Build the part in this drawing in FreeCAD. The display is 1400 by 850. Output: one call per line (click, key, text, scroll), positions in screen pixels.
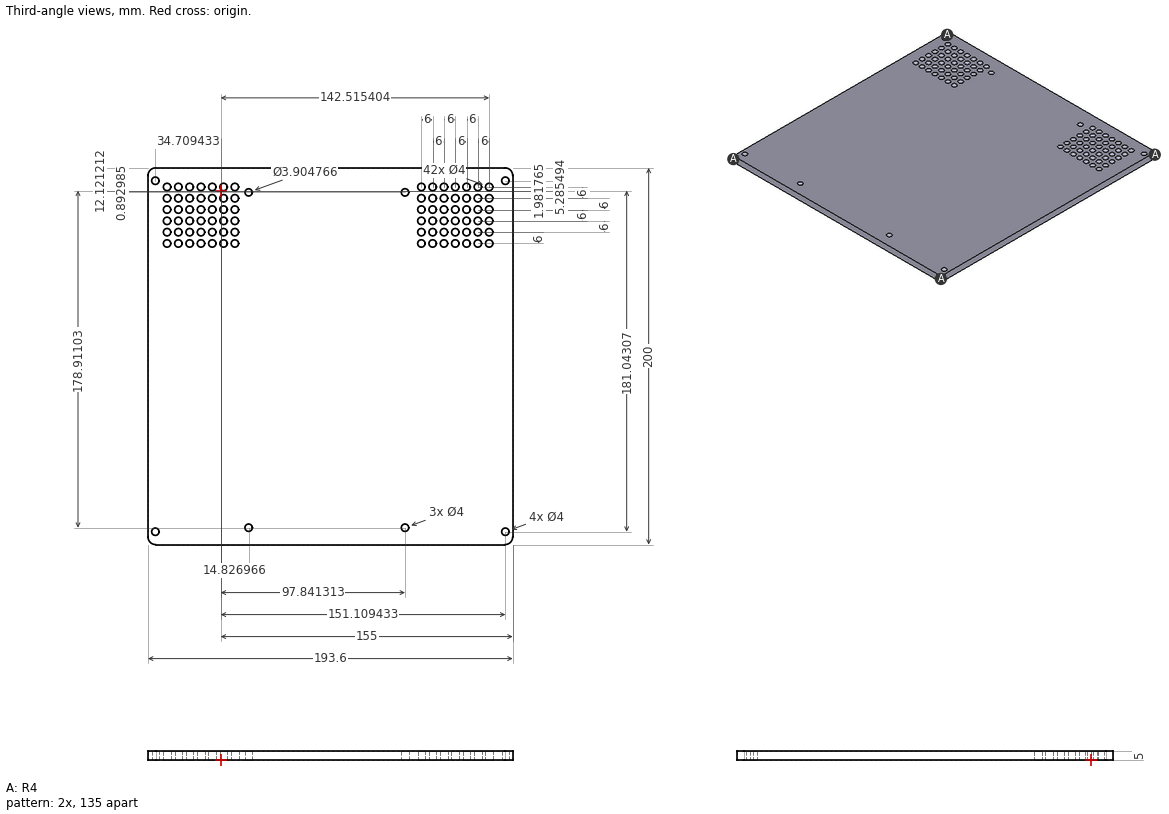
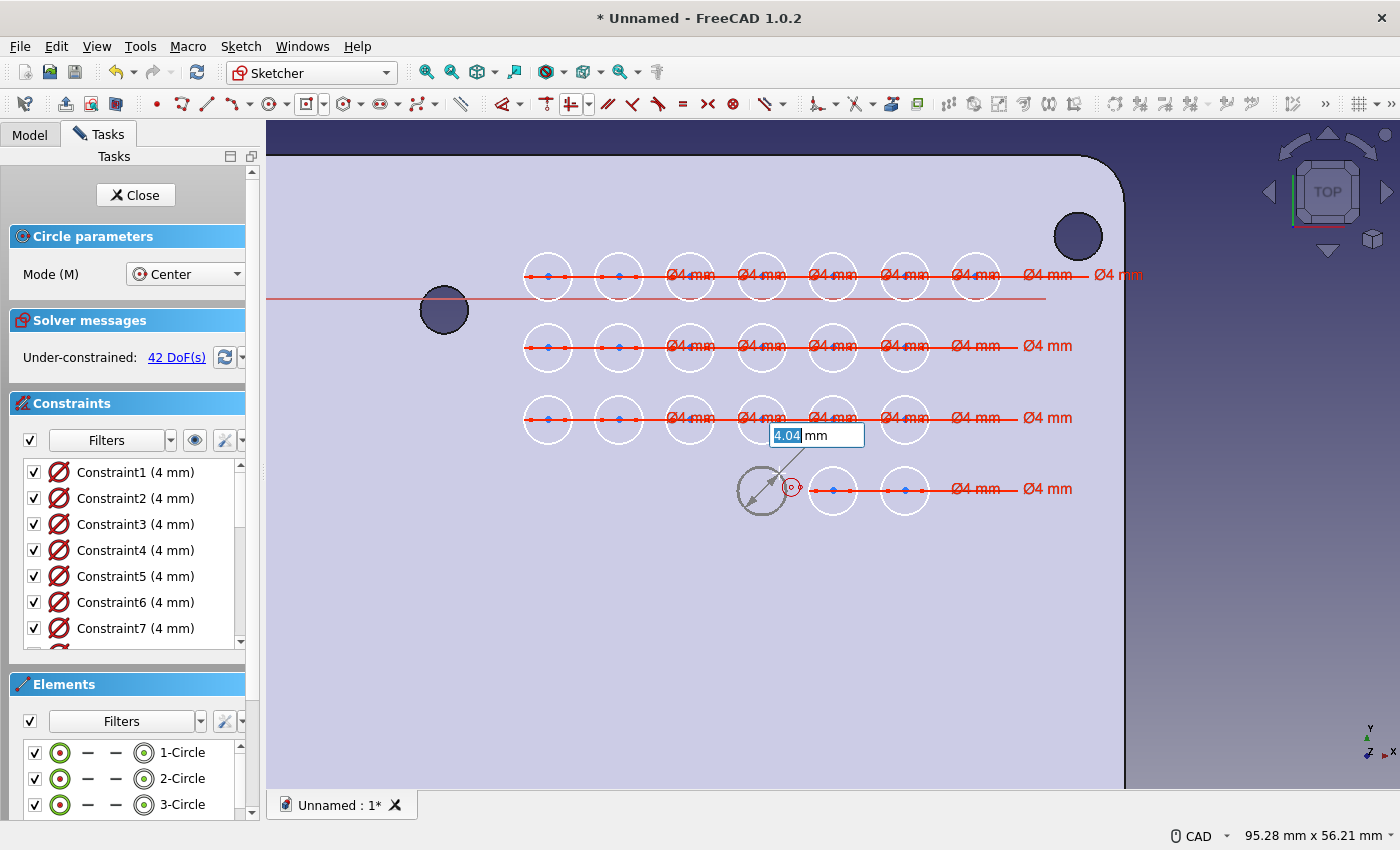
text(4)
key(Return)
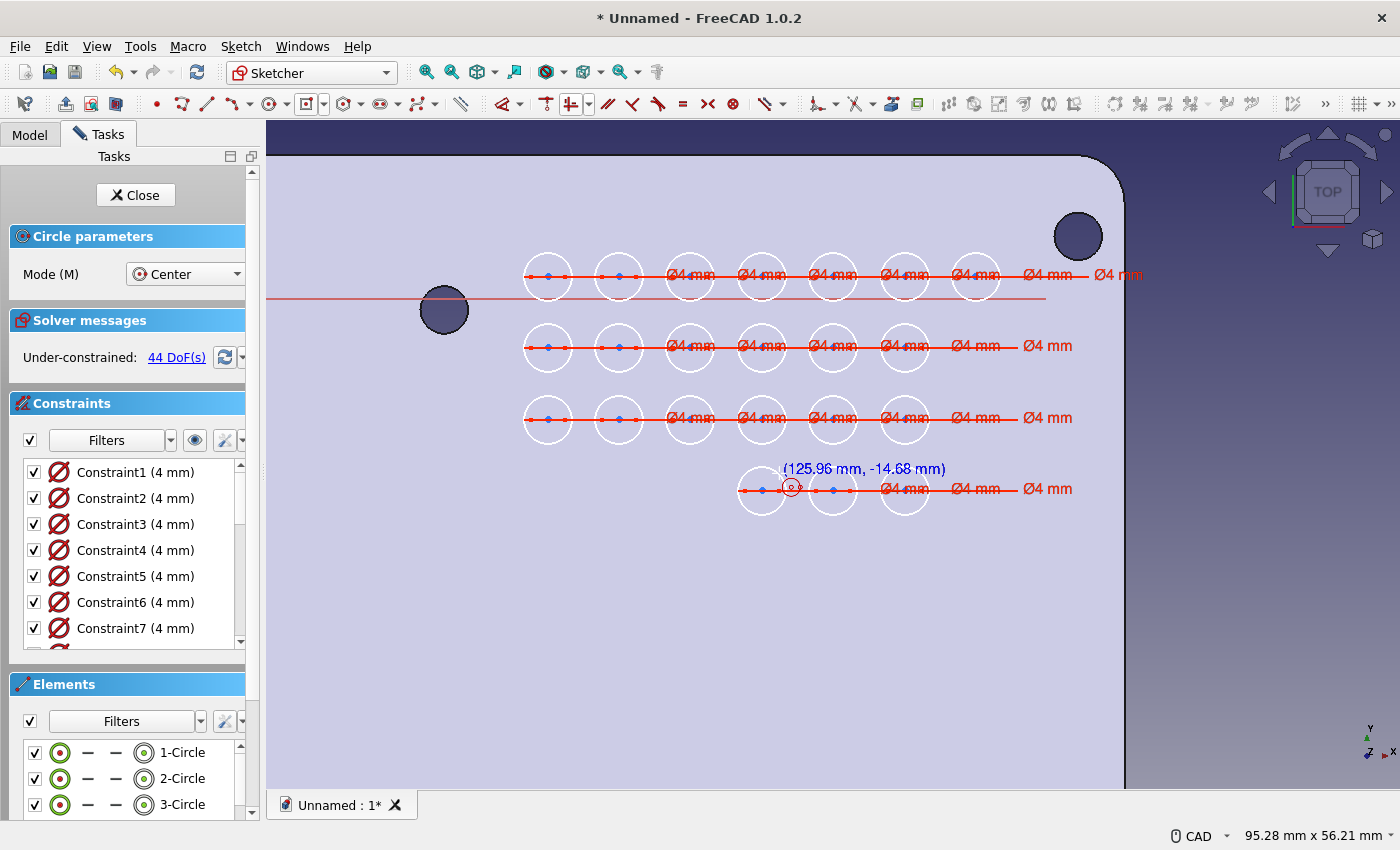
click(690, 490)
move(707, 473)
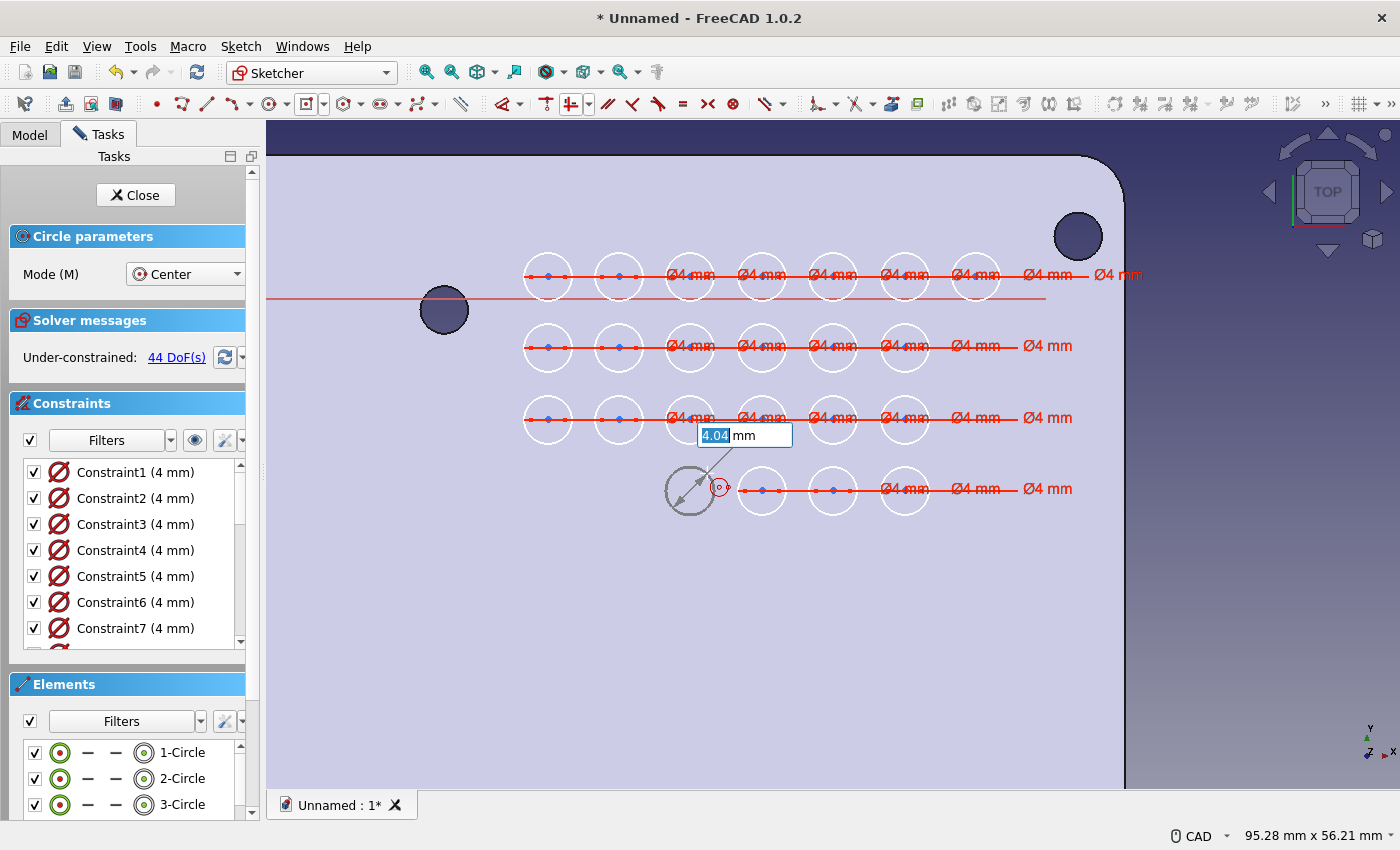
text(4)
key(Return)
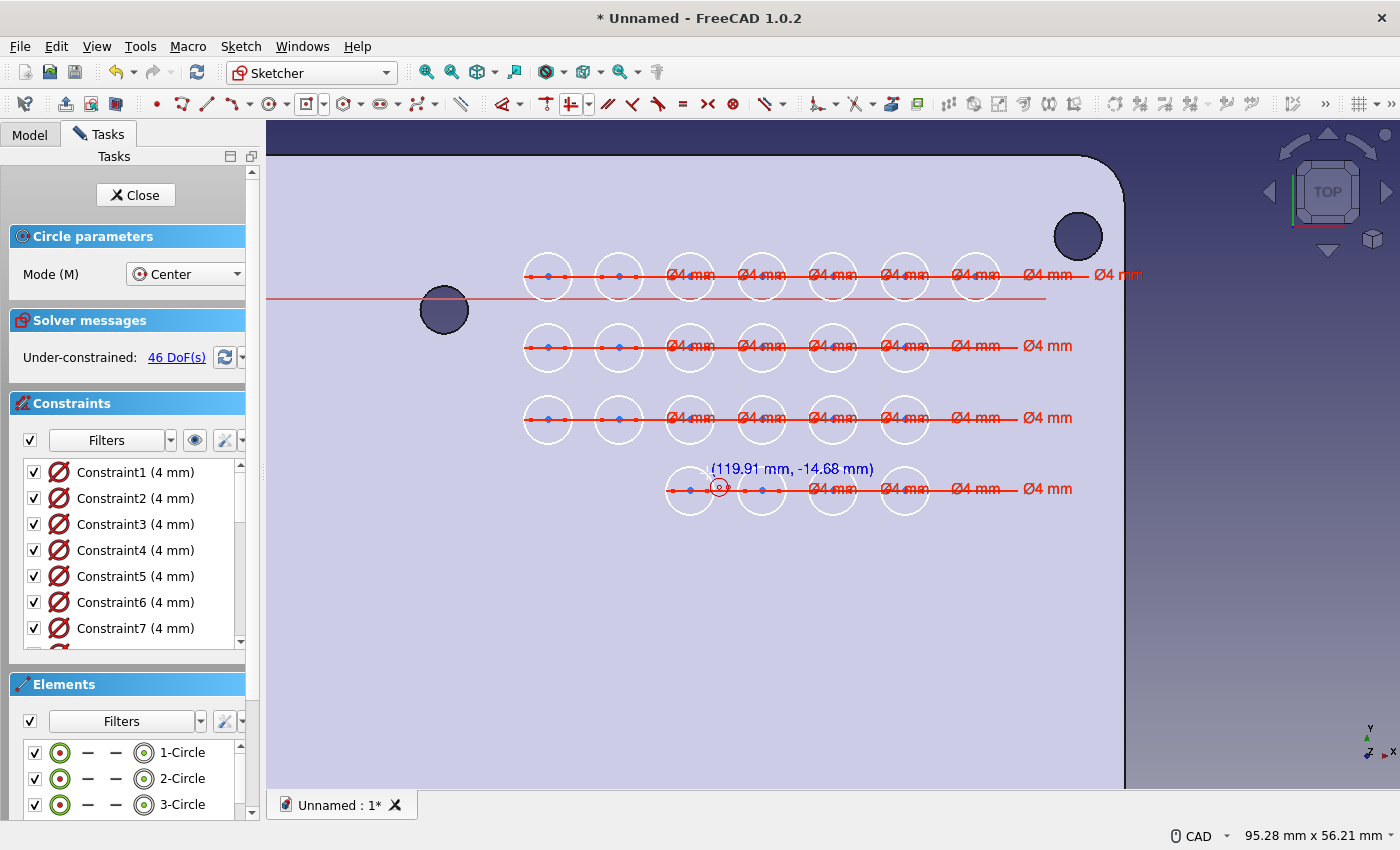
click(619, 490)
move(636, 473)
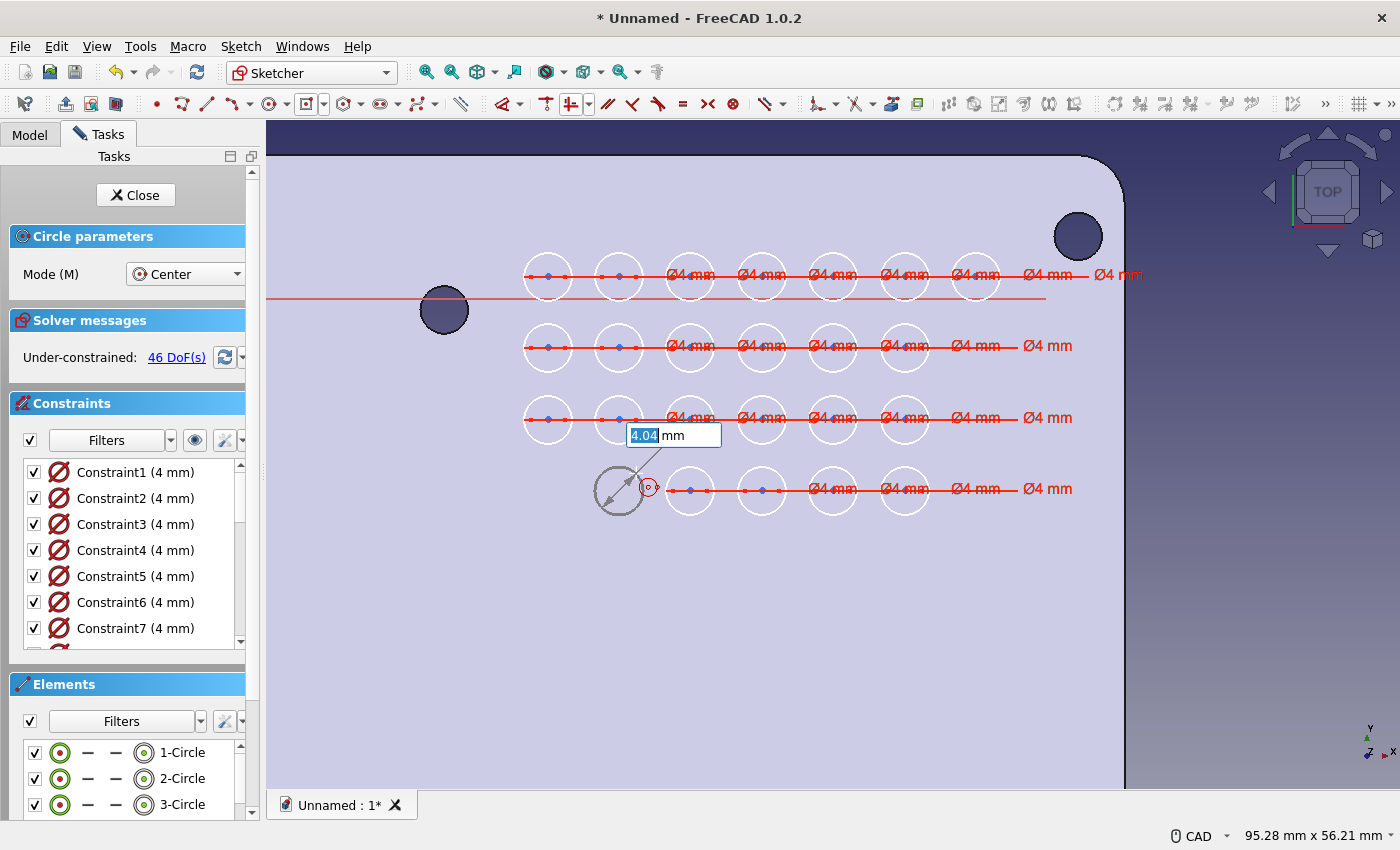
text(4)
key(Return)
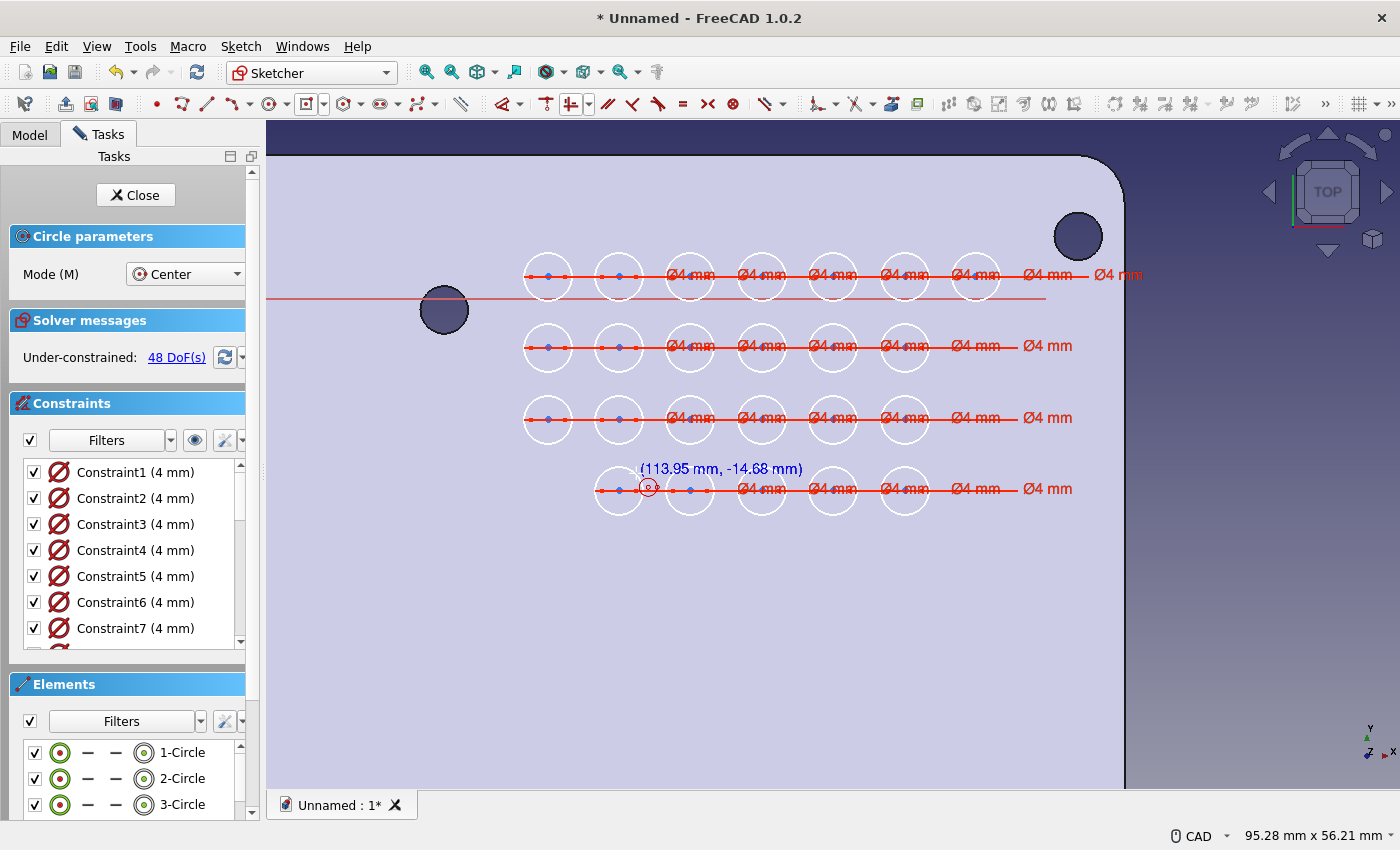
click(548, 490)
move(564, 473)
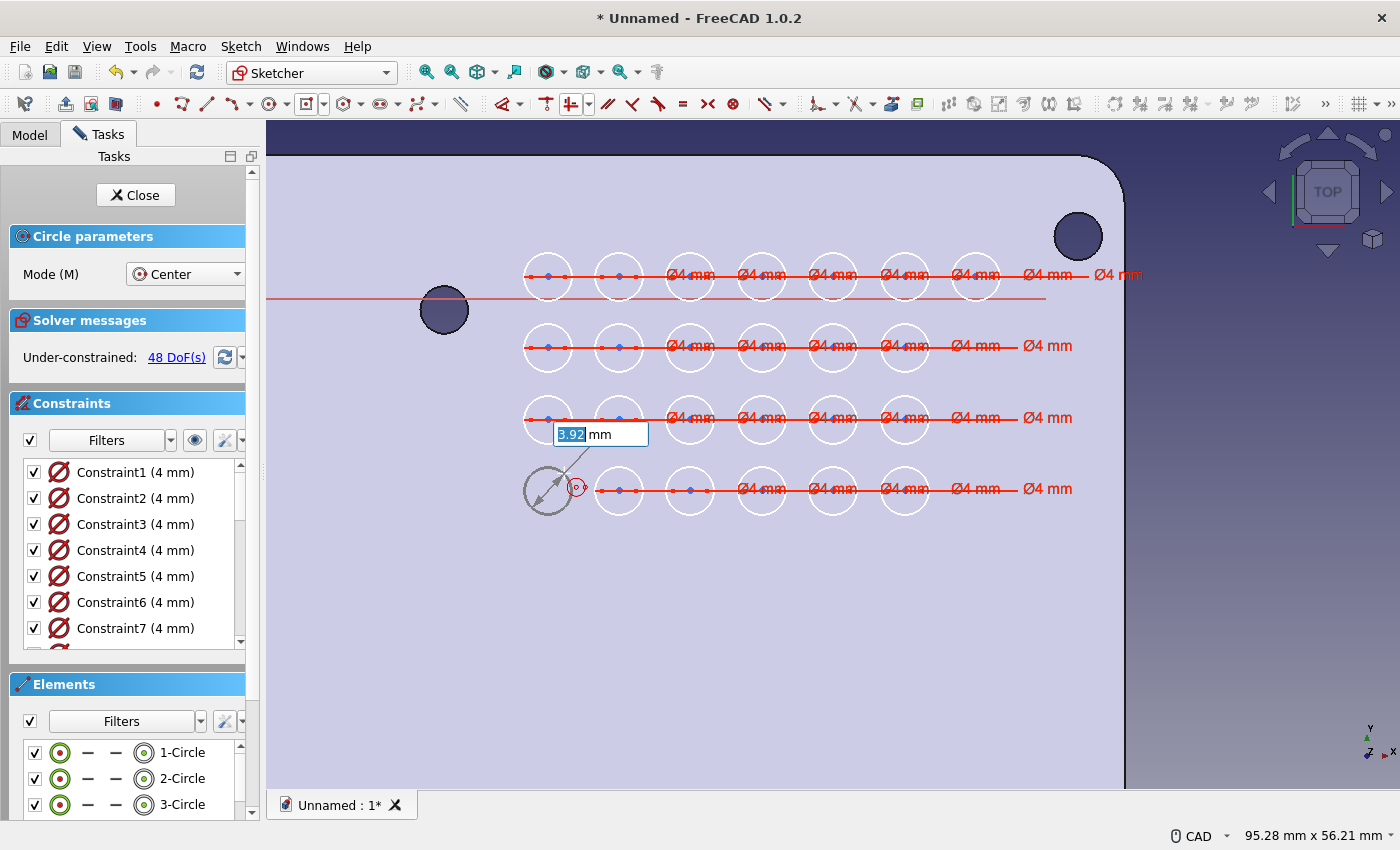
text(4)
key(Return)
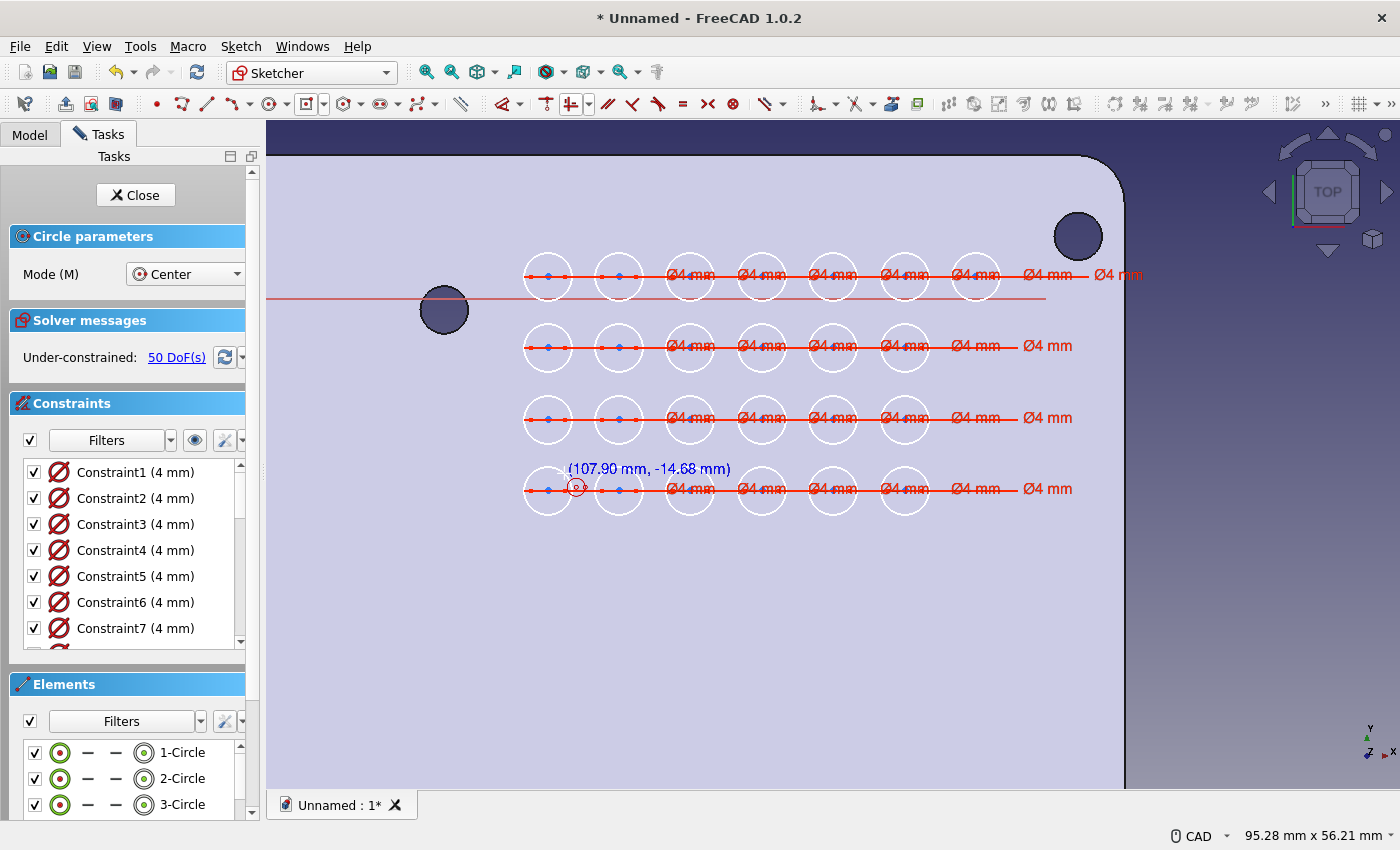
click(905, 561)
move(921, 545)